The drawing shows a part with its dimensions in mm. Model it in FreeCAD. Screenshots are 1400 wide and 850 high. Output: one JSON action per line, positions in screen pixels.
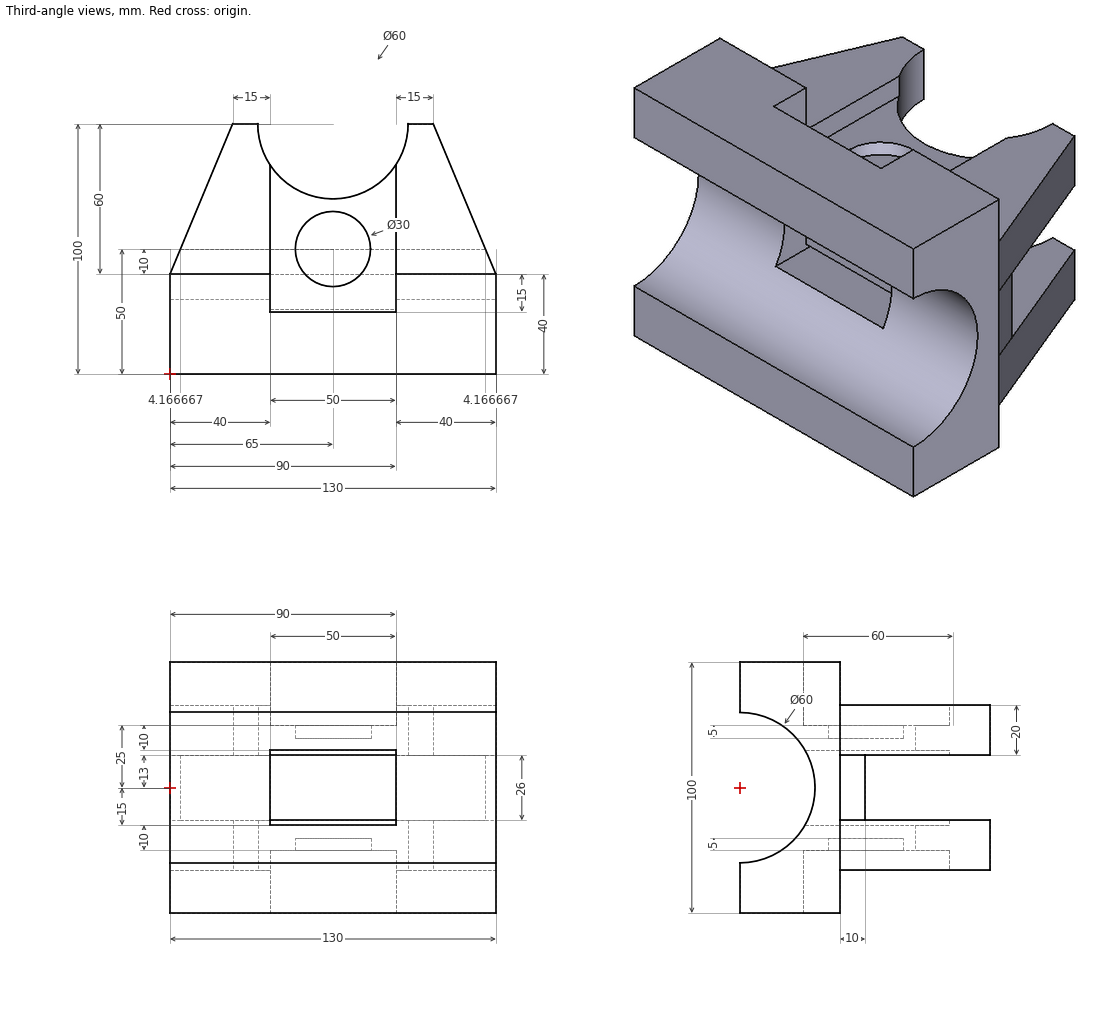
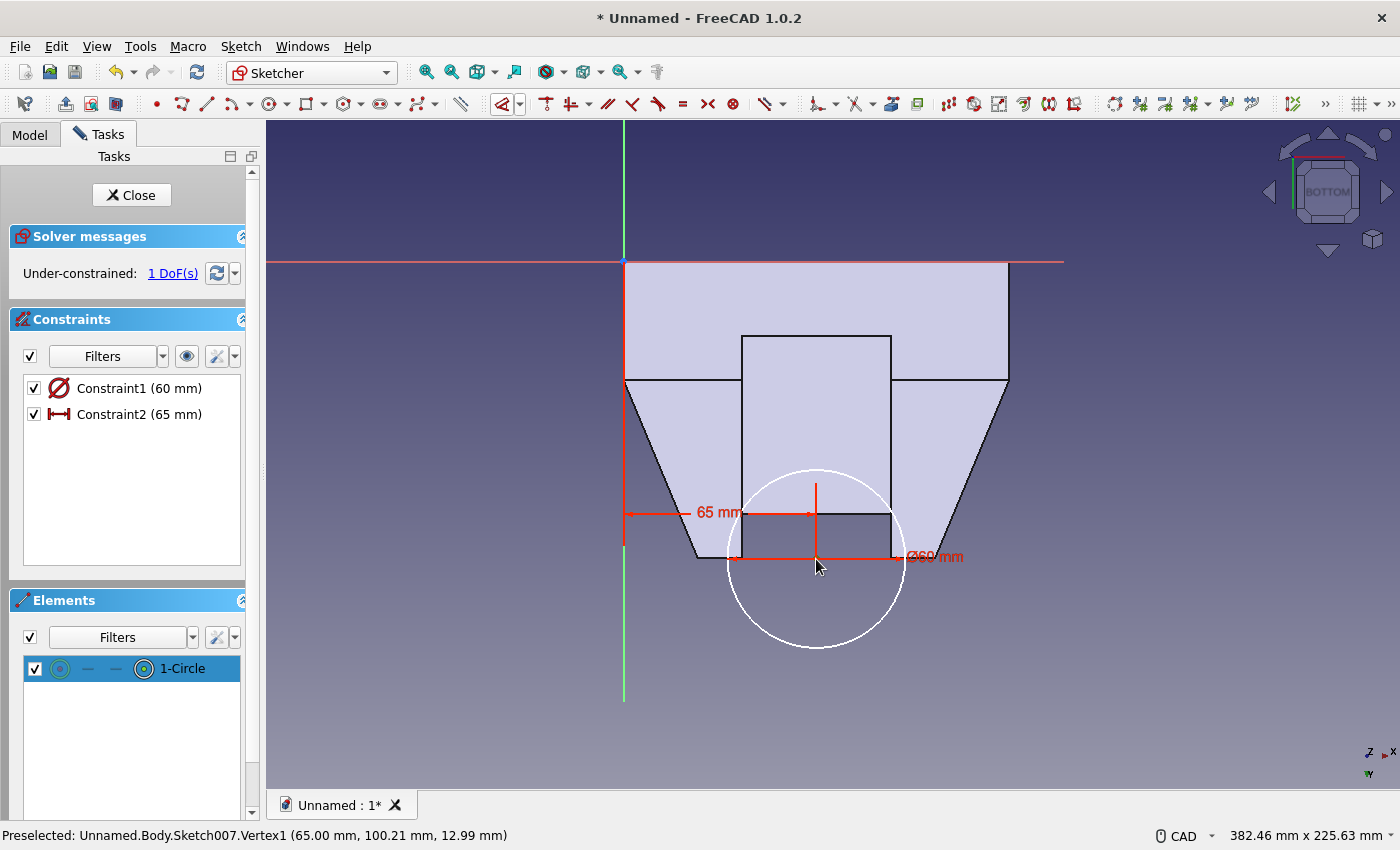
{"action": "left_click", "coordinate": [520, 104]}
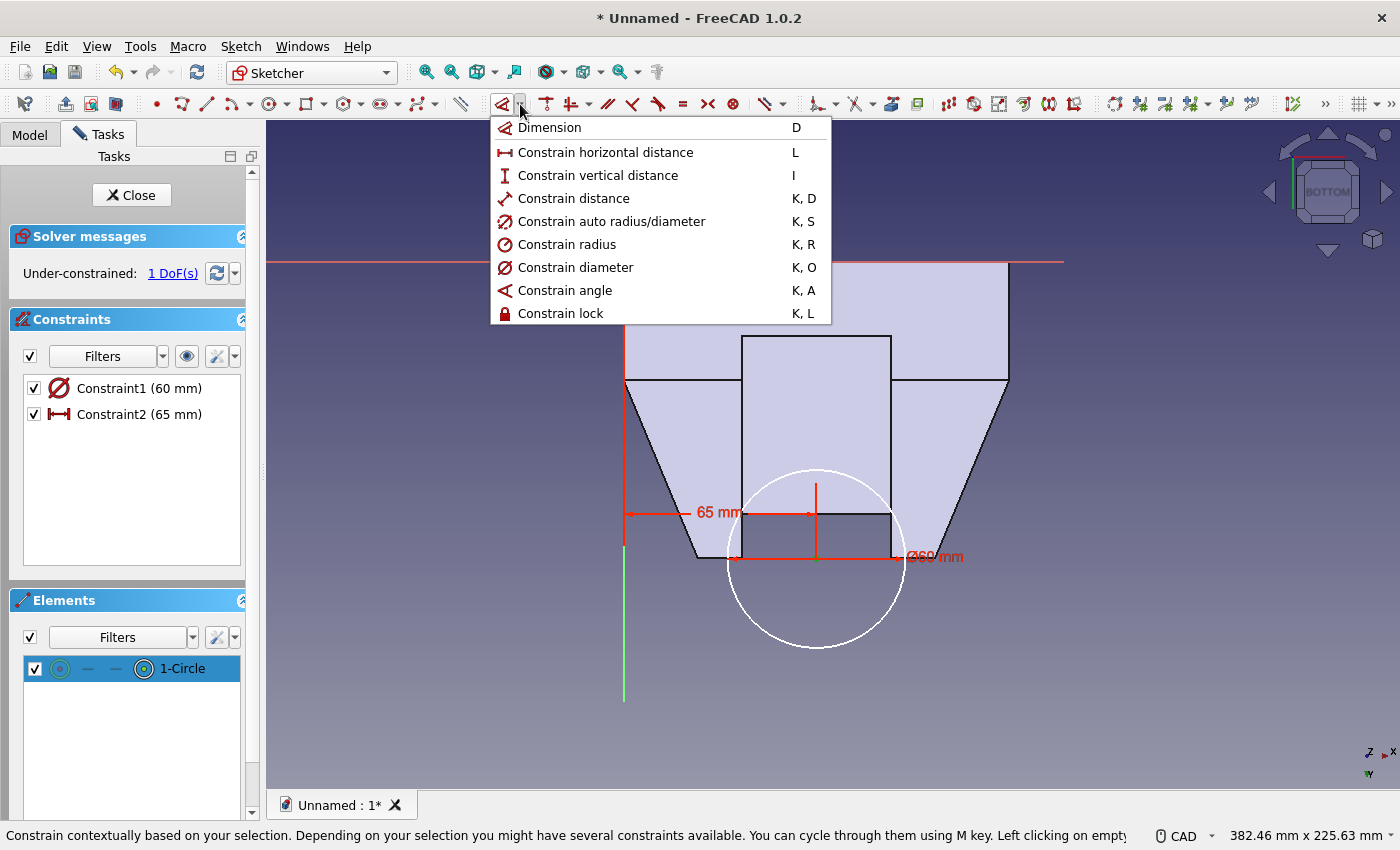
{"action": "left_click", "coordinate": [661, 176]}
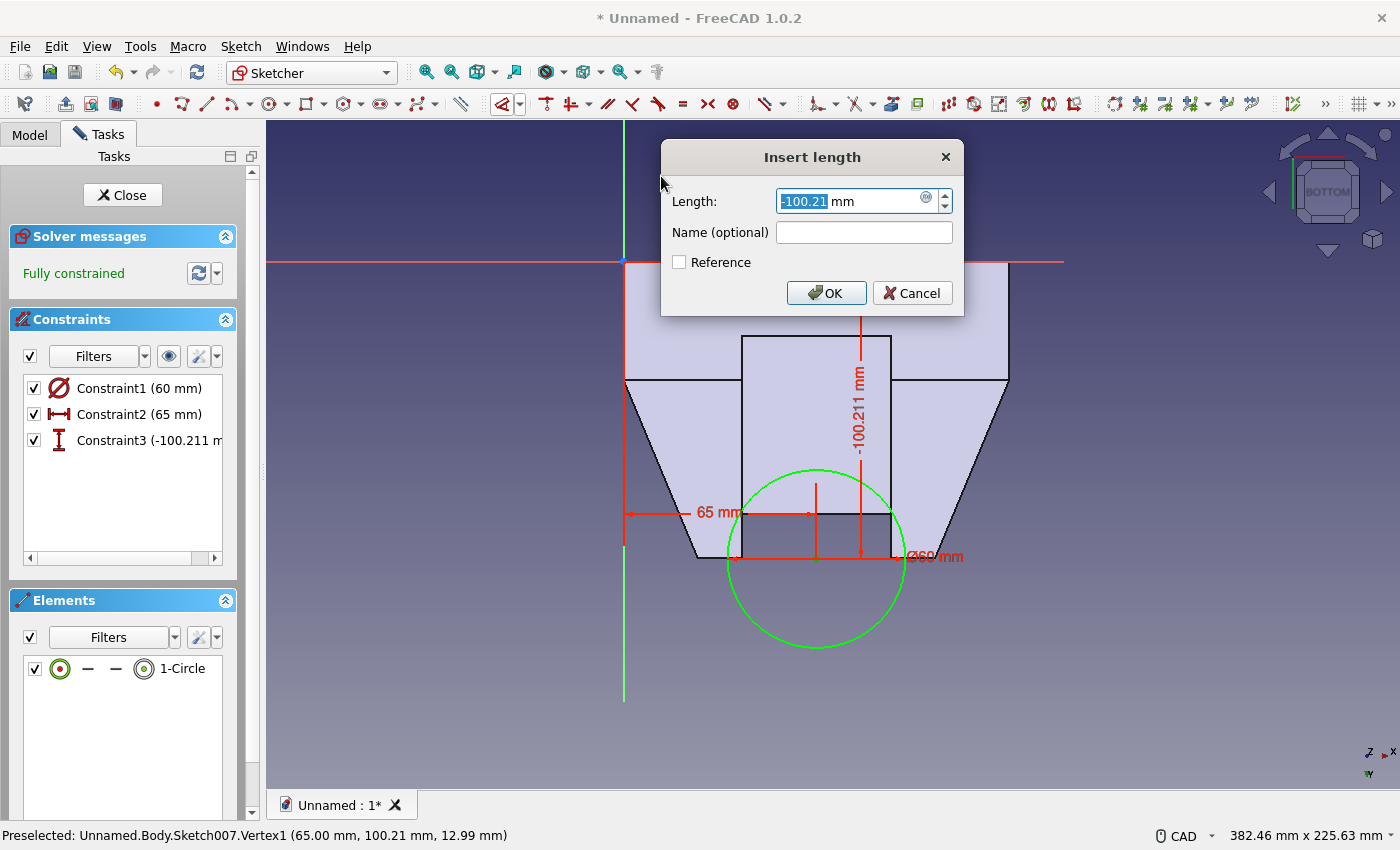
{"action": "type", "text": "-100"}
{"action": "key", "text": "Return"}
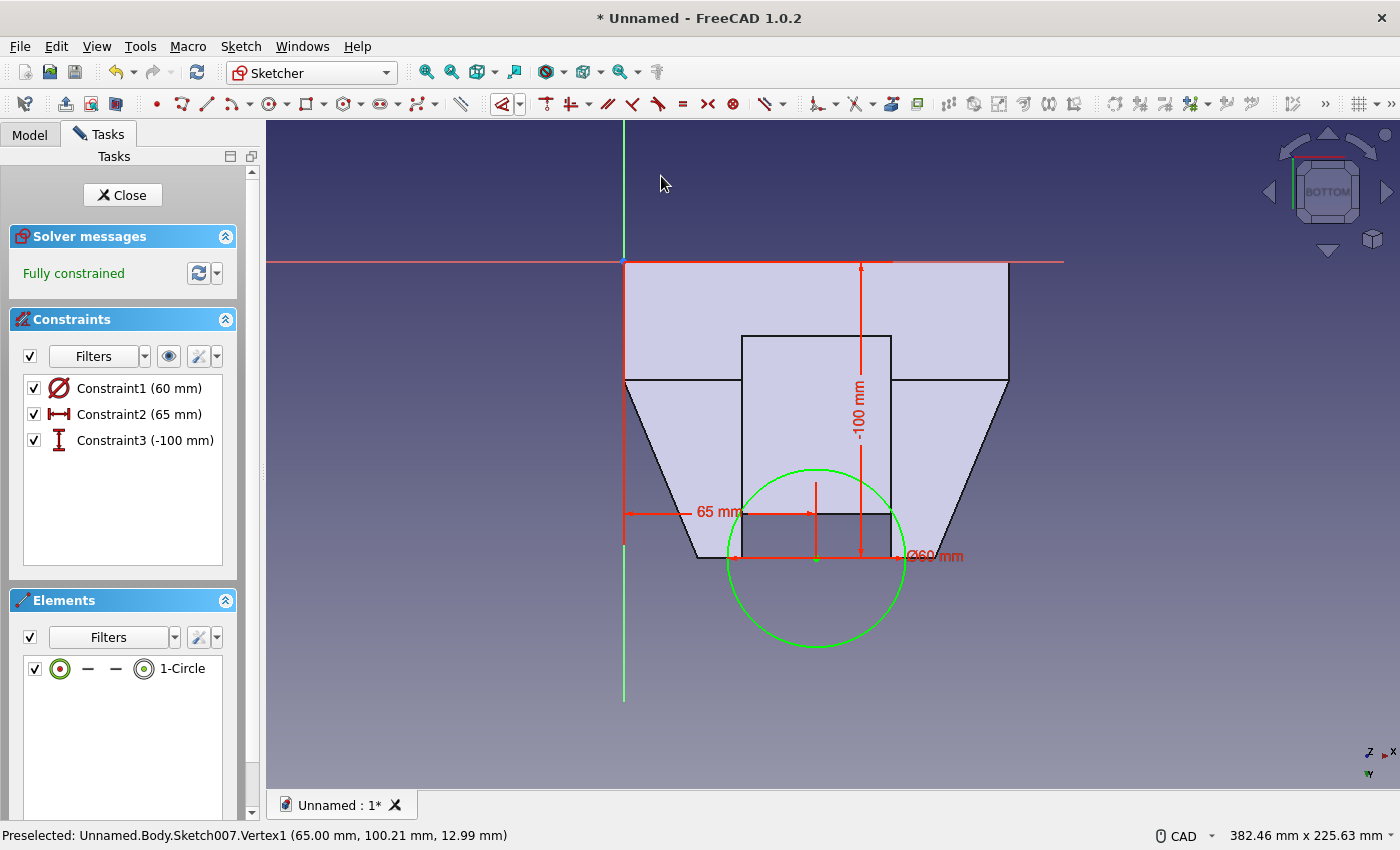
{"action": "left_click", "coordinate": [123, 195]}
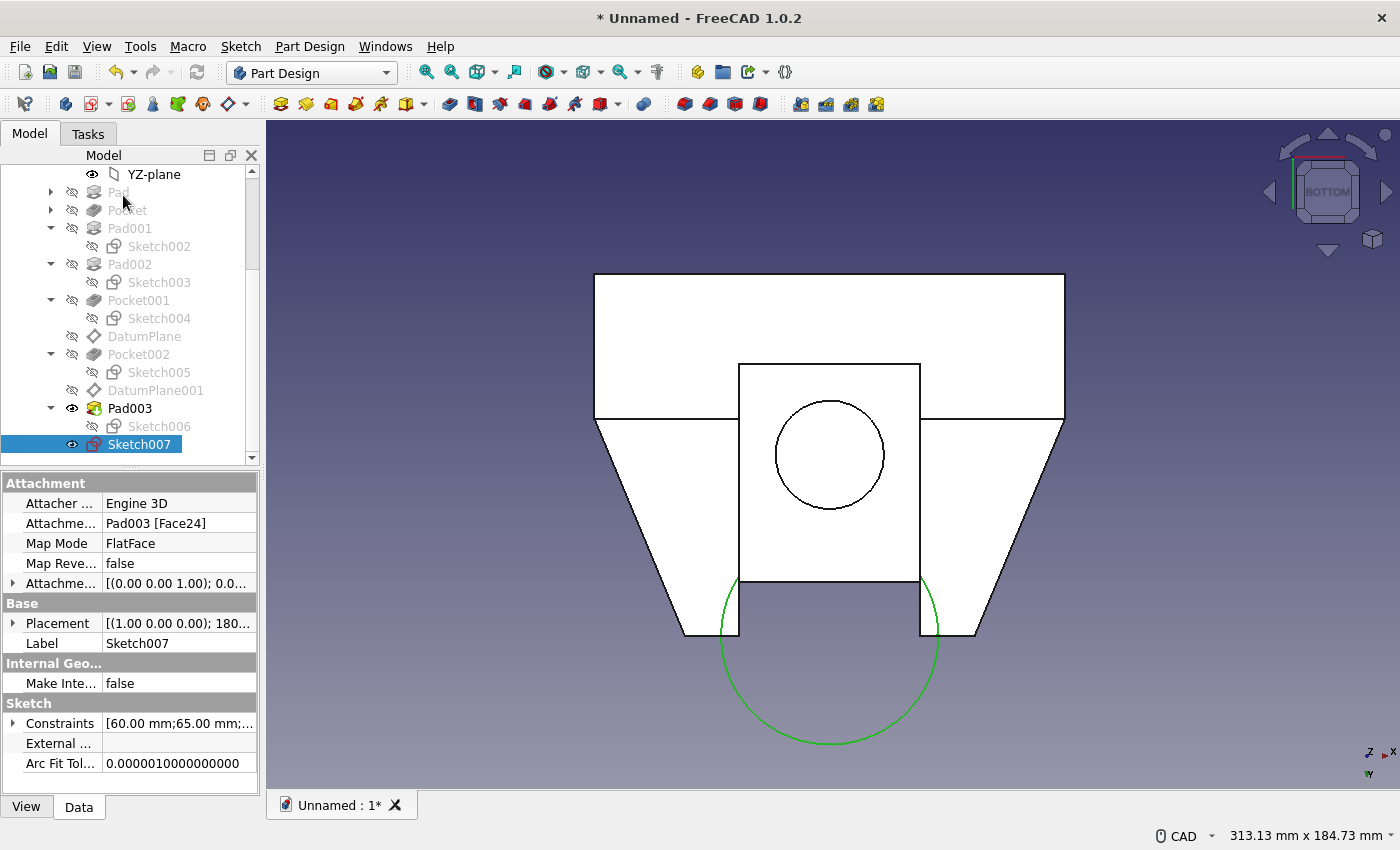
{"action": "left_click", "coordinate": [450, 104]}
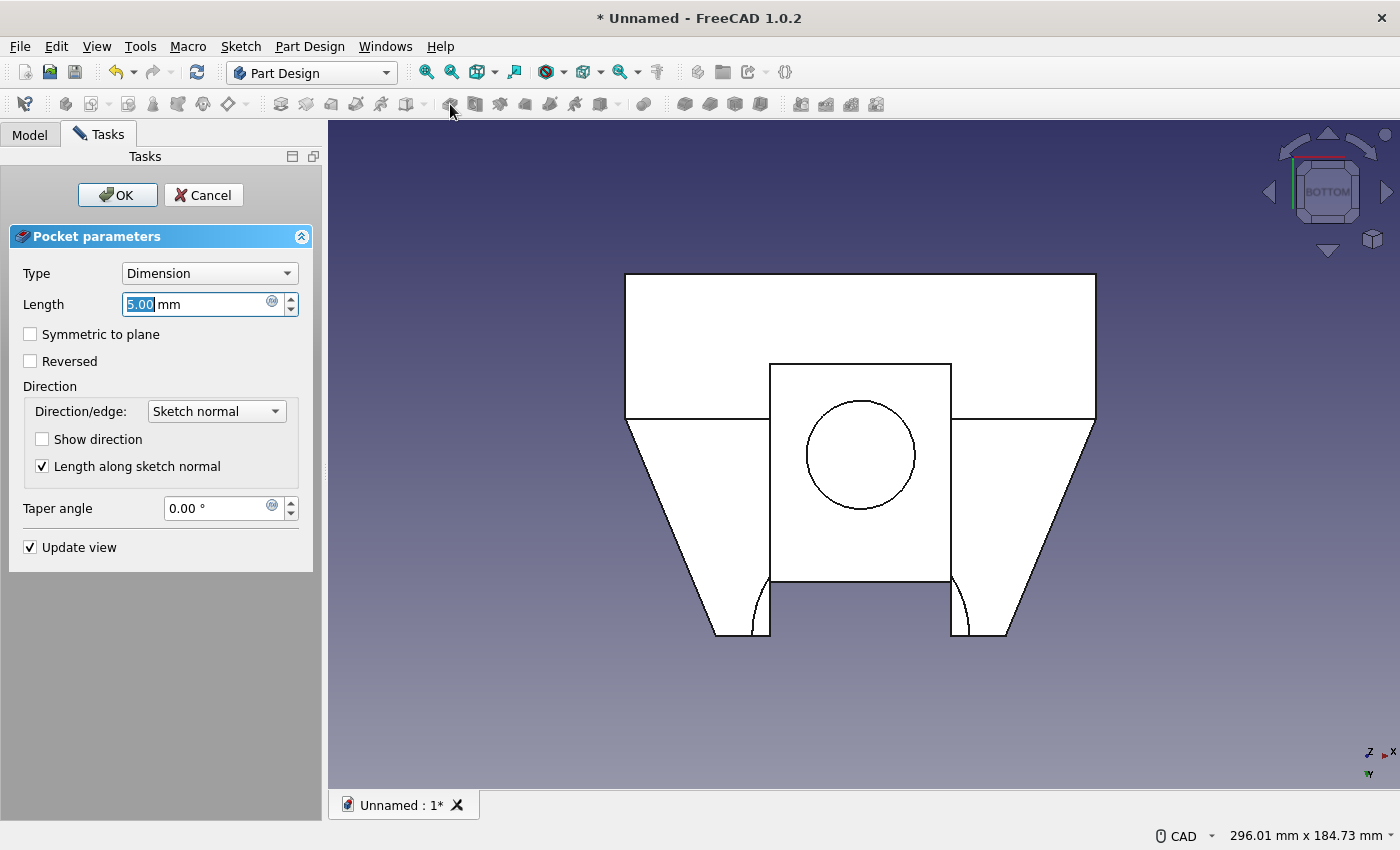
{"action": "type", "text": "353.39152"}
{"action": "key", "text": "Tab"}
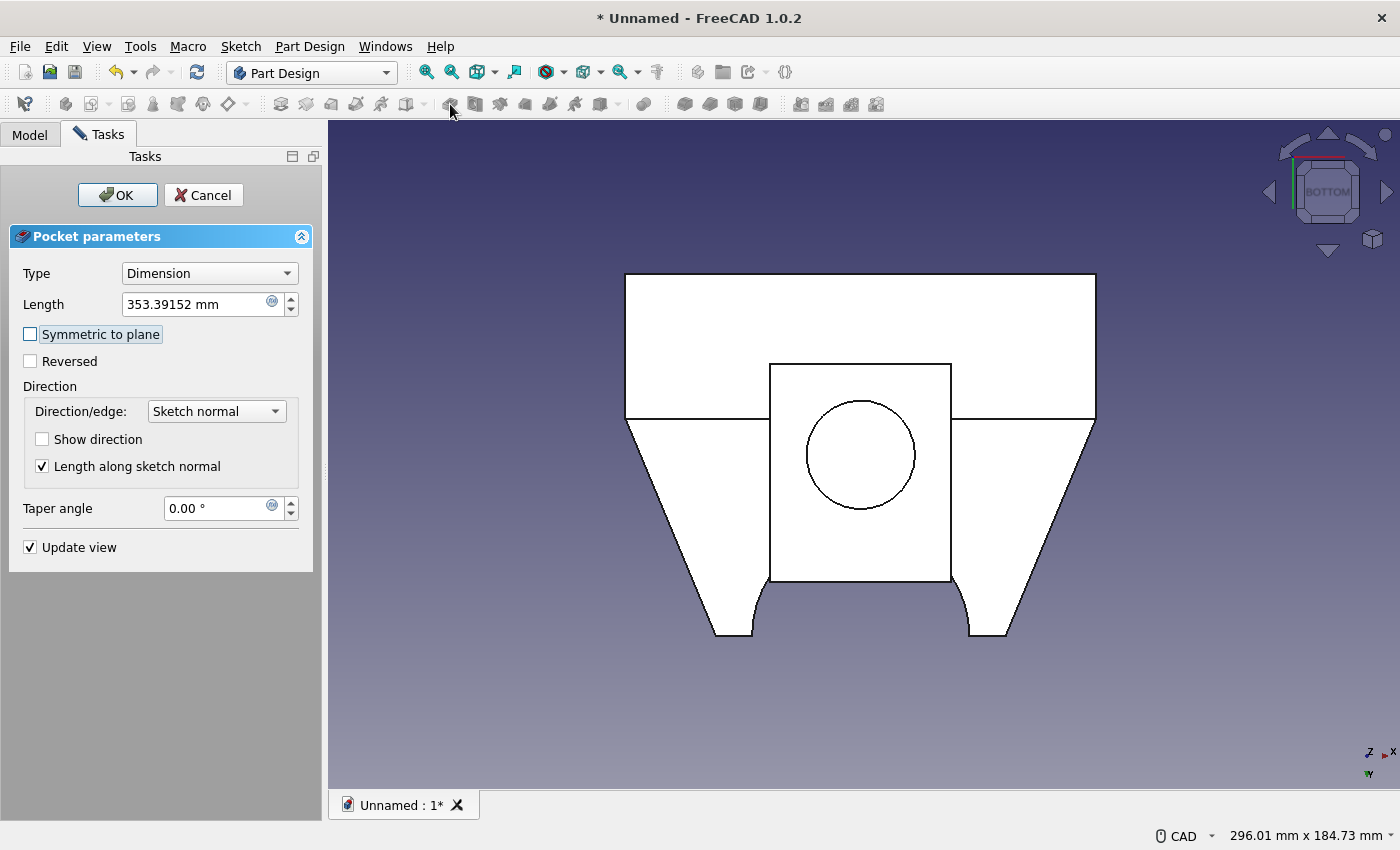
{"action": "left_click", "coordinate": [31, 334]}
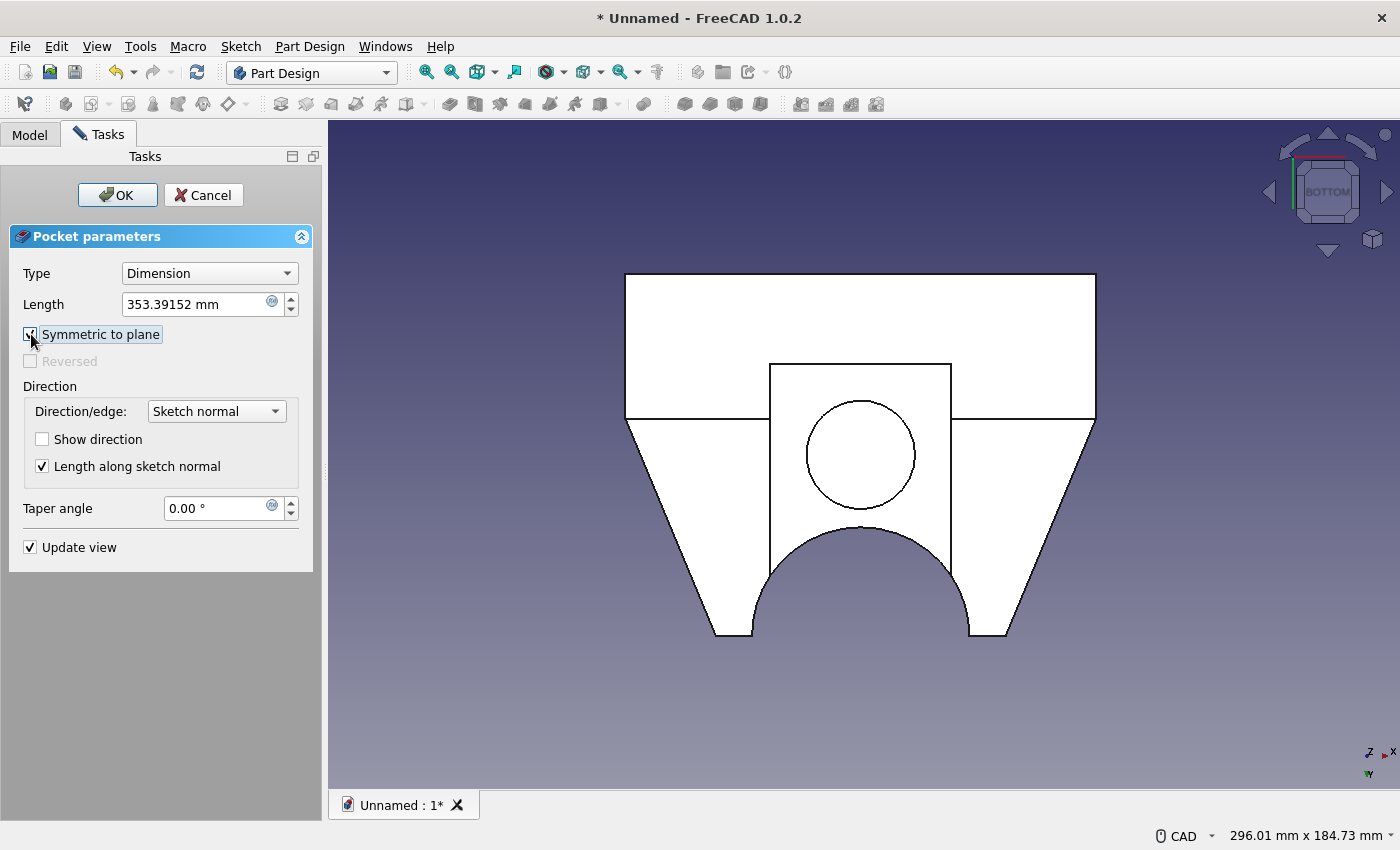
{"action": "left_click", "coordinate": [118, 195]}